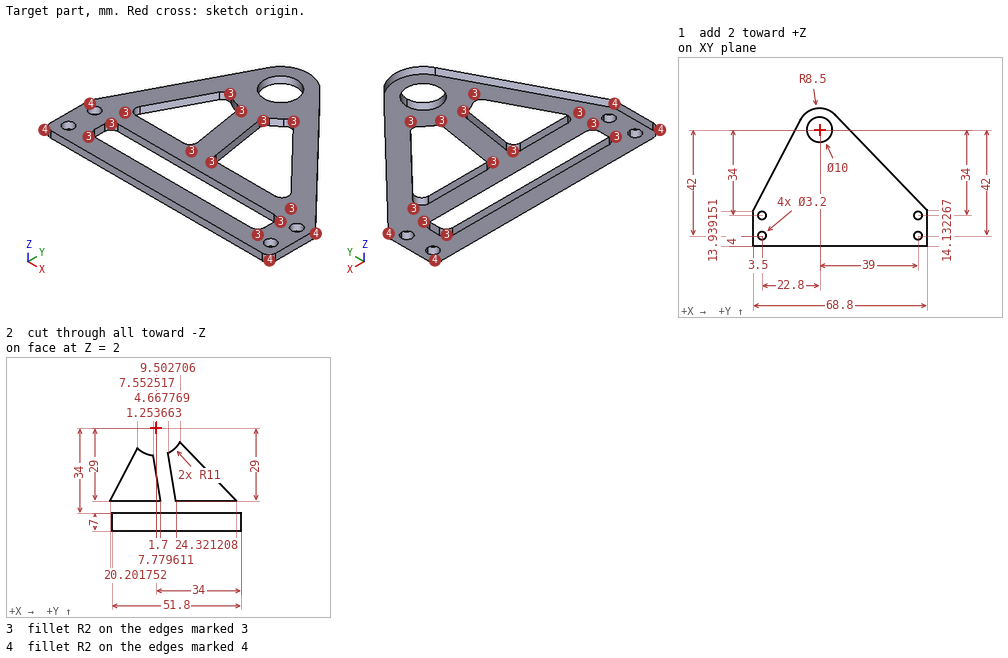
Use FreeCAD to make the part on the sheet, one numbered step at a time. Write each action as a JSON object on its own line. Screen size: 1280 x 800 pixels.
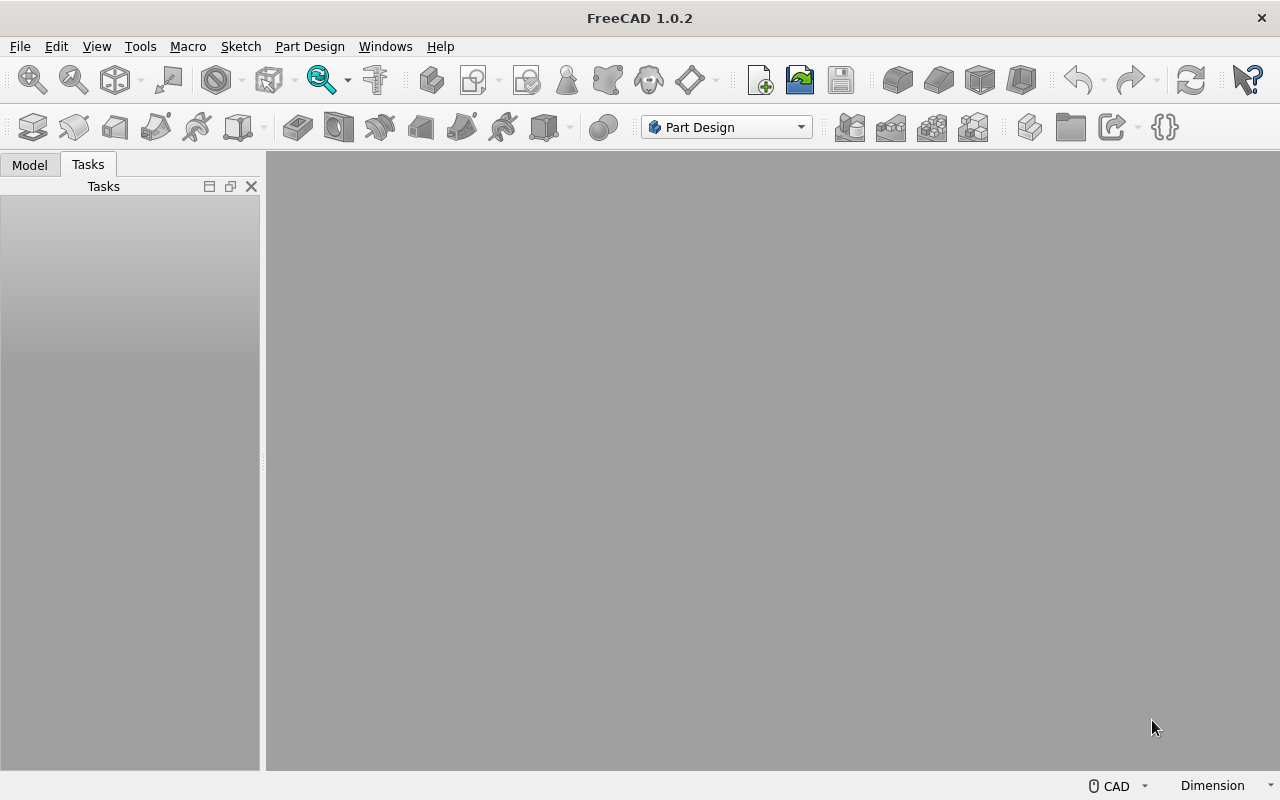
{"action": "left_click", "coordinate": [759, 80]}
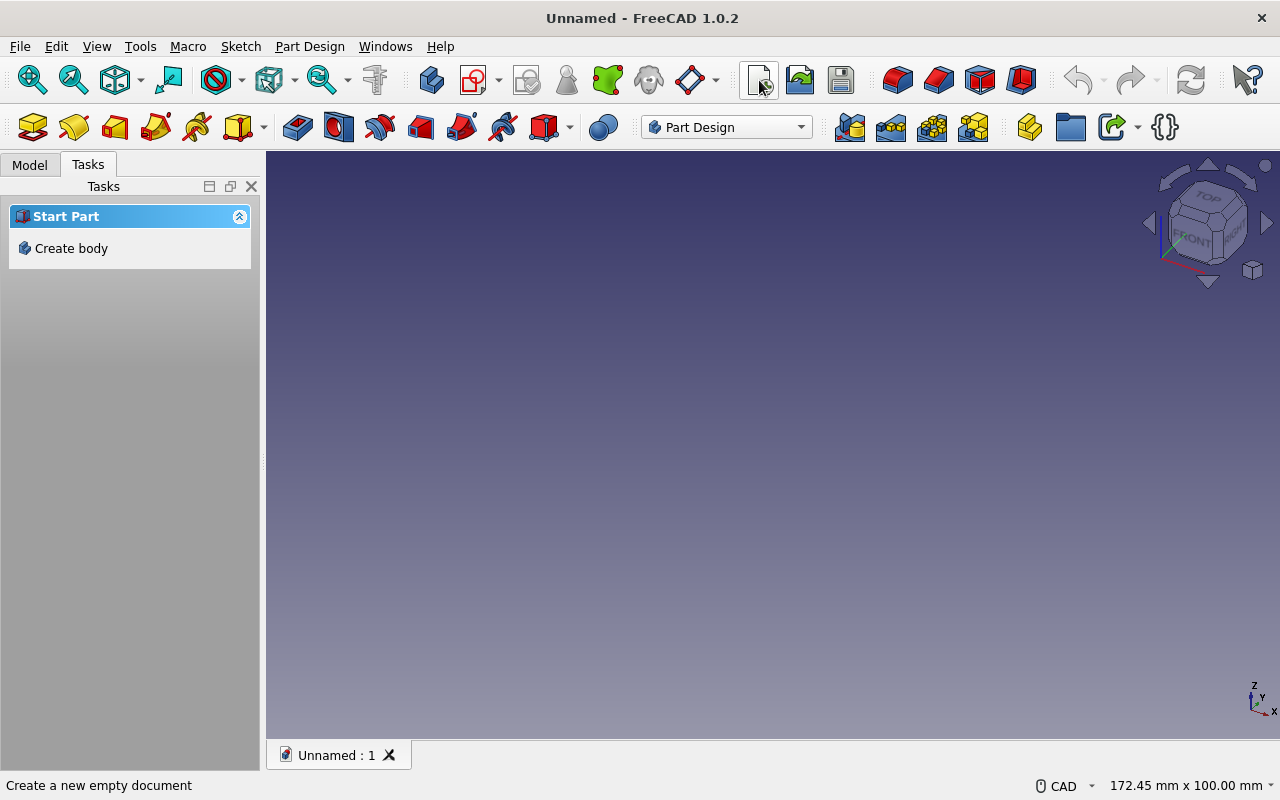
{"action": "left_click", "coordinate": [472, 80]}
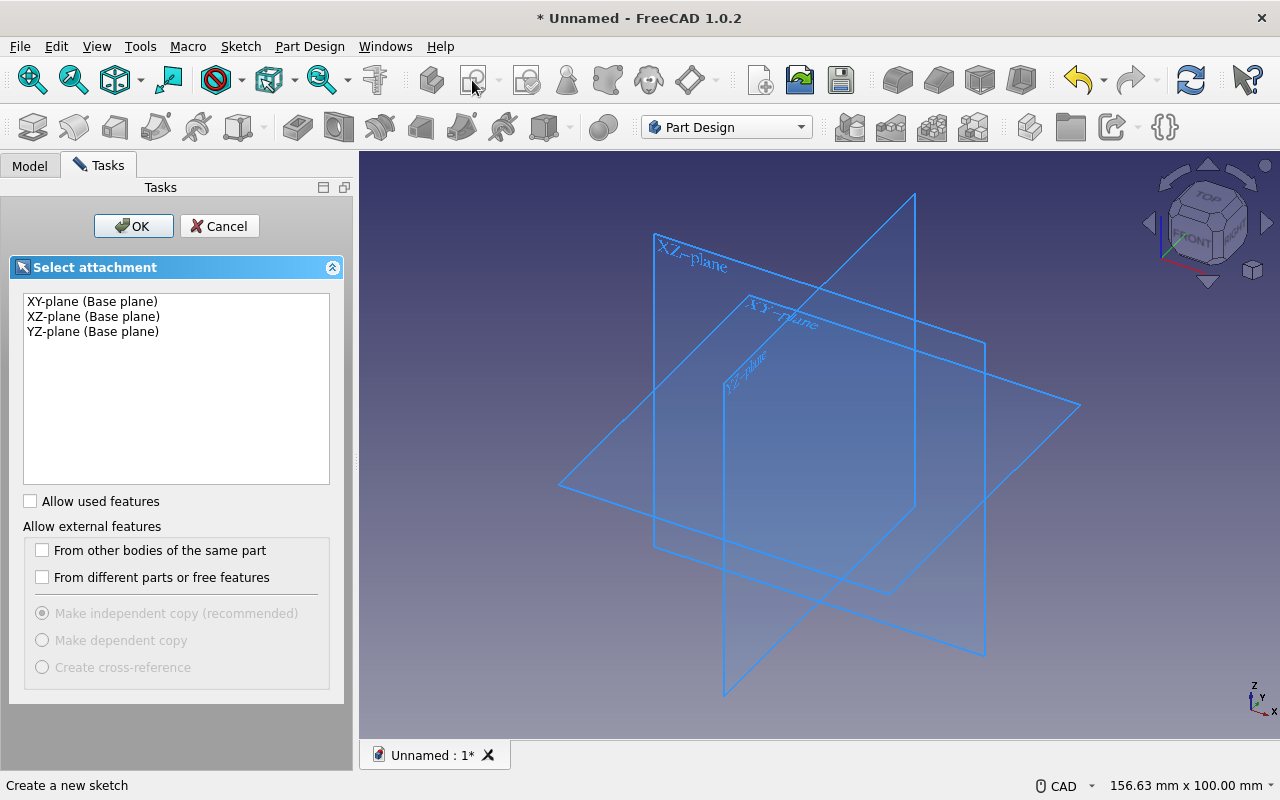
{"action": "left_click", "coordinate": [84, 302]}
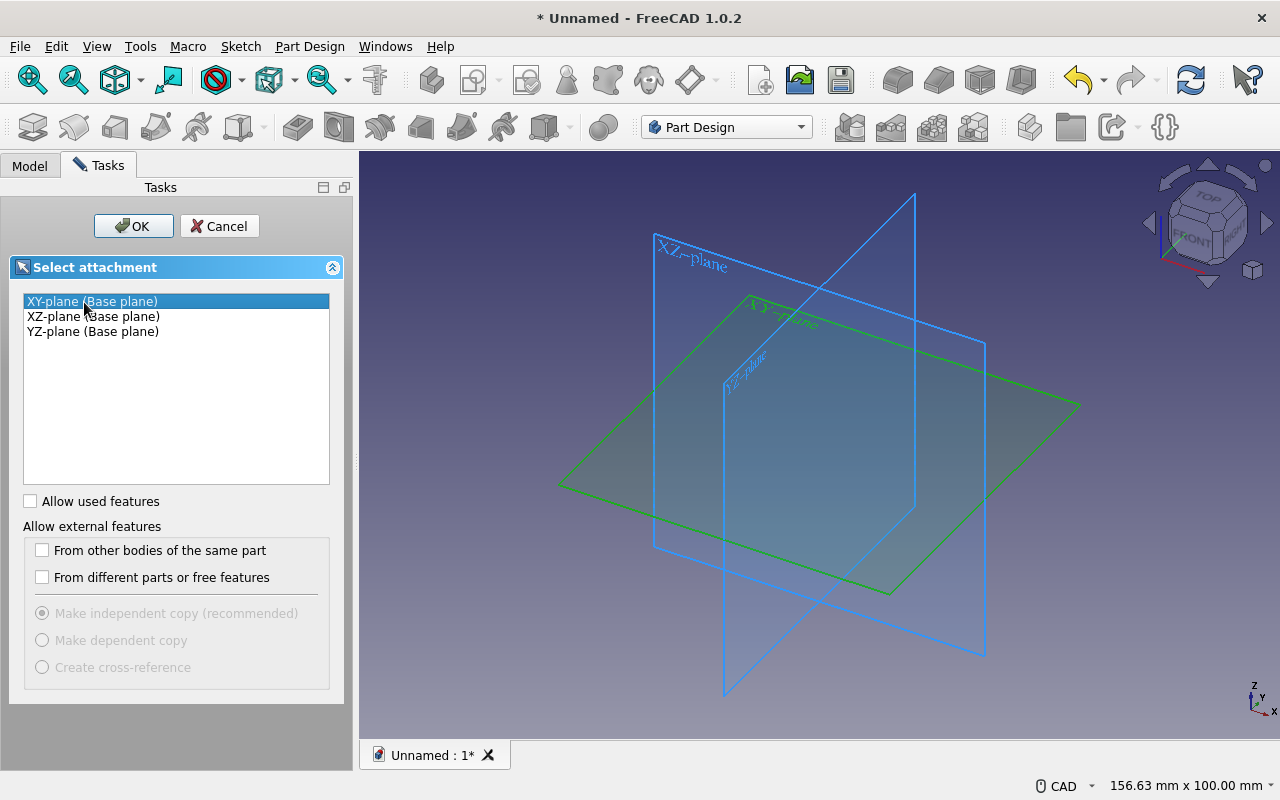
{"action": "left_click", "coordinate": [134, 226]}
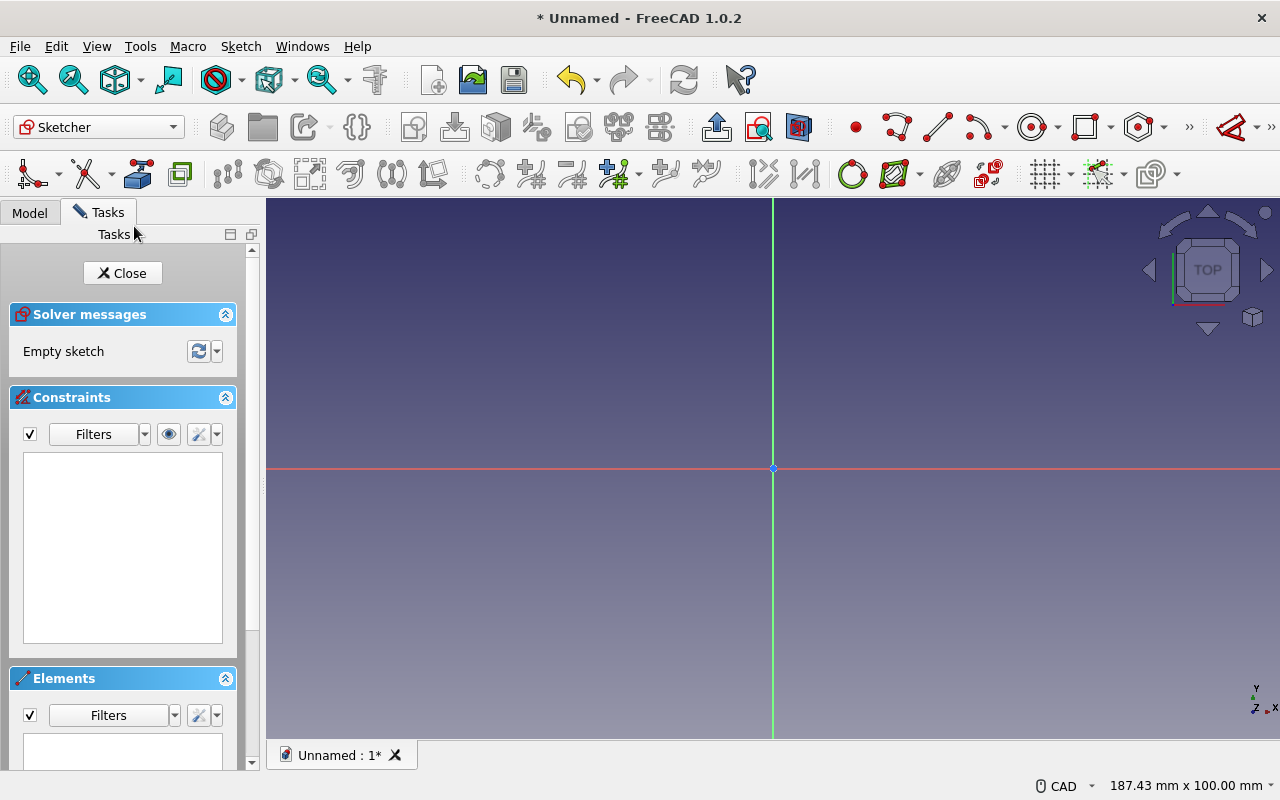
{"action": "scroll", "coordinate": [294, 226], "scroll_direction": "down", "scroll_amount": 1}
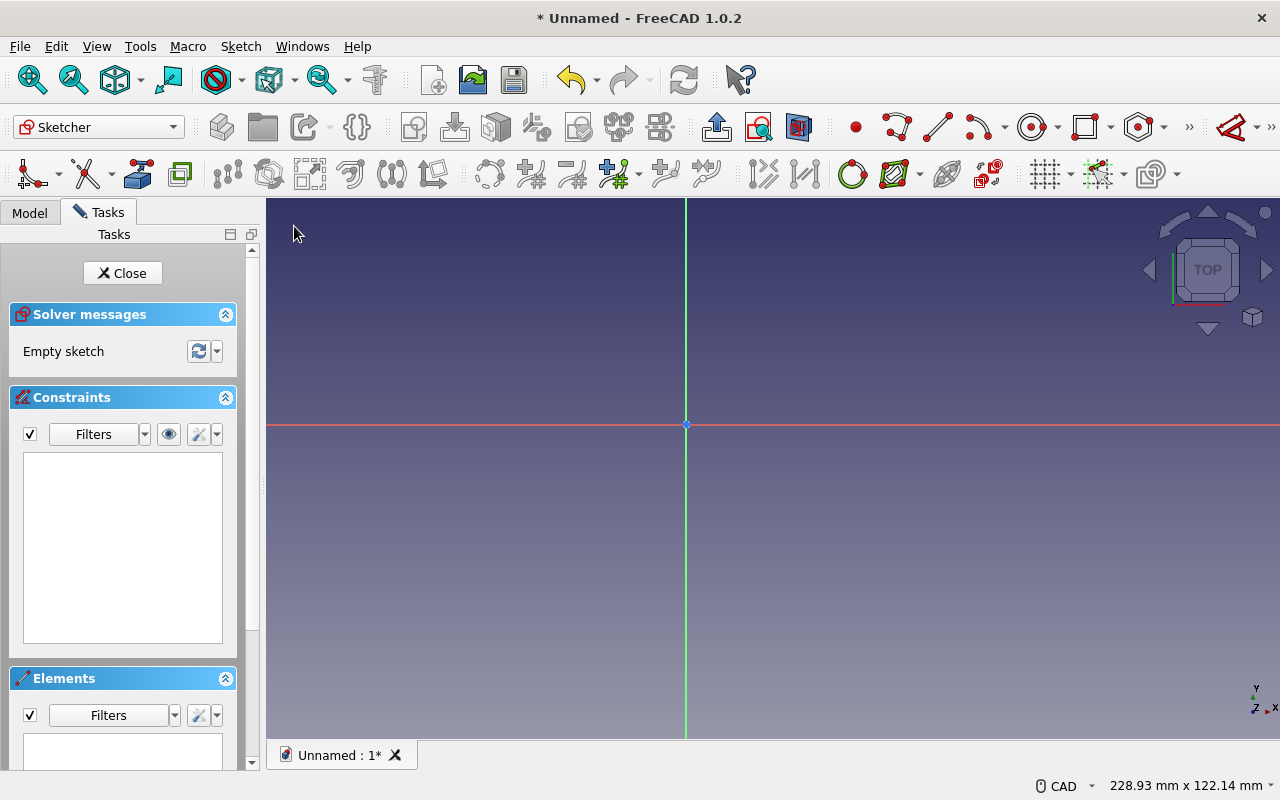
{"action": "scroll", "coordinate": [758, 588], "scroll_direction": "up", "scroll_amount": 2}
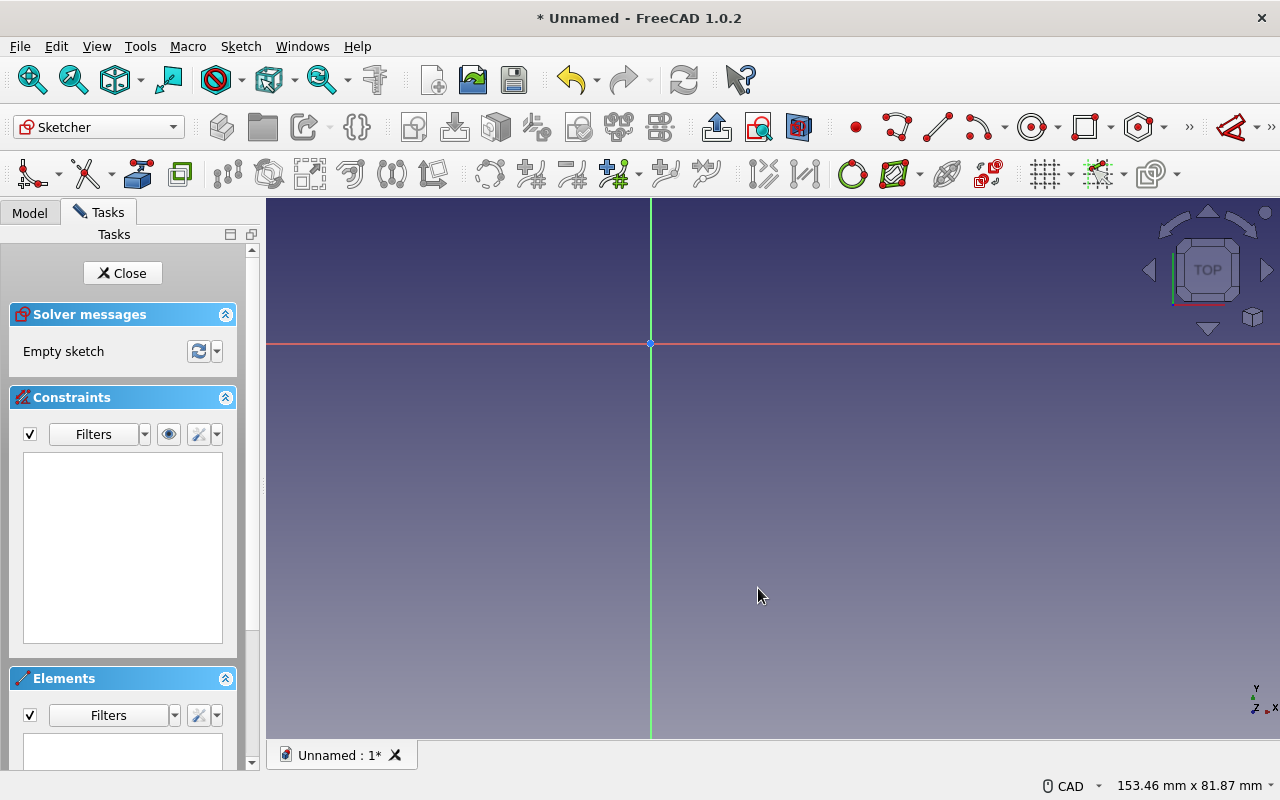
{"action": "key", "text": "g m"}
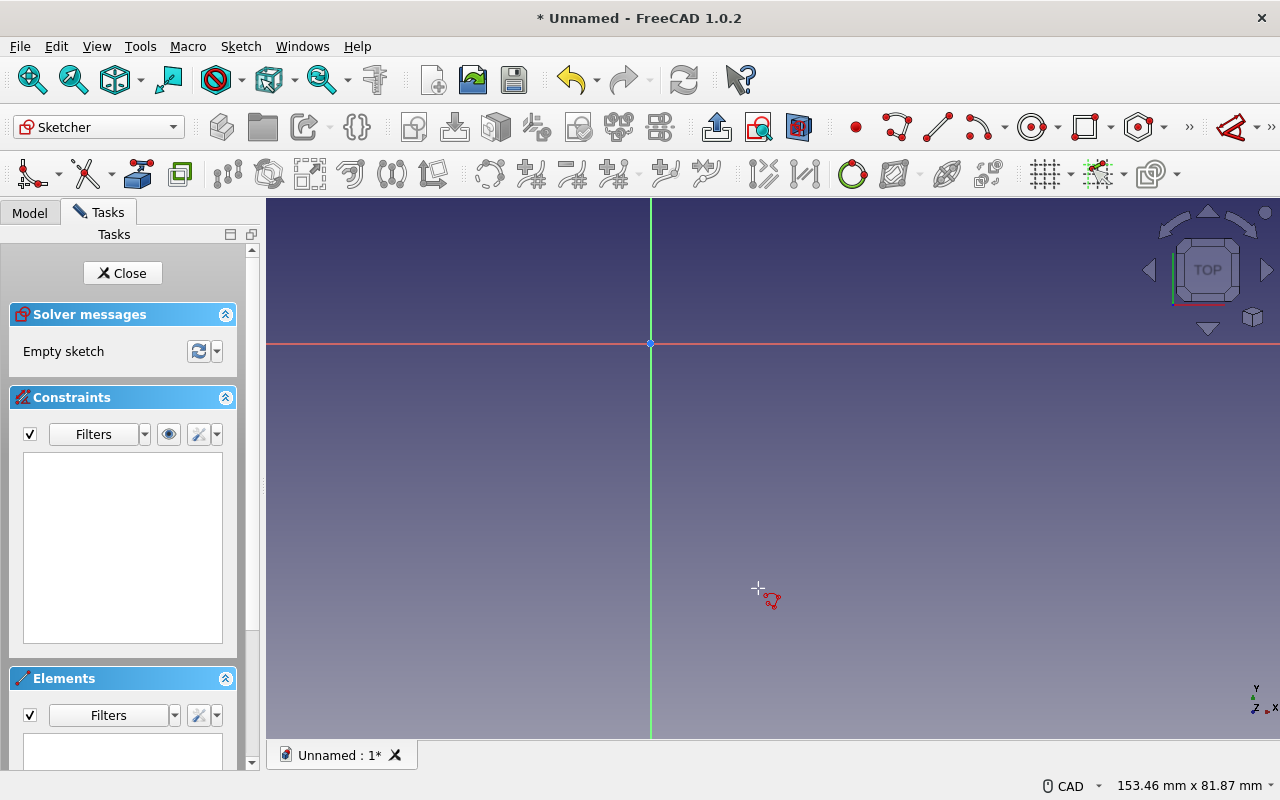
{"action": "left_click", "coordinate": [601, 318]}
{"action": "left_click", "coordinate": [477, 556]}
{"action": "left_click", "coordinate": [477, 648]}
{"action": "left_click", "coordinate": [931, 648]}
{"action": "left_click", "coordinate": [931, 554]}
{"action": "left_click", "coordinate": [691, 305]}
{"action": "right_click", "coordinate": [691, 305]}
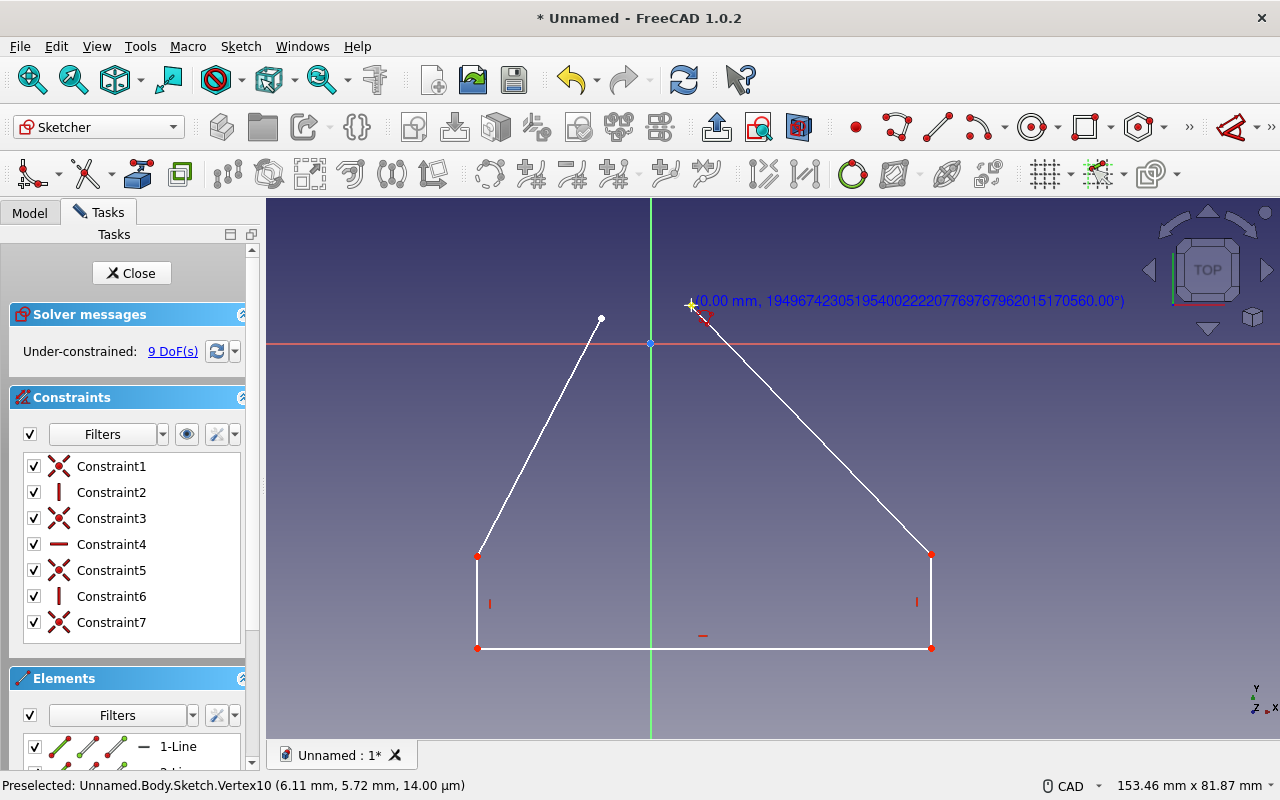
{"action": "key", "text": "g 3 a"}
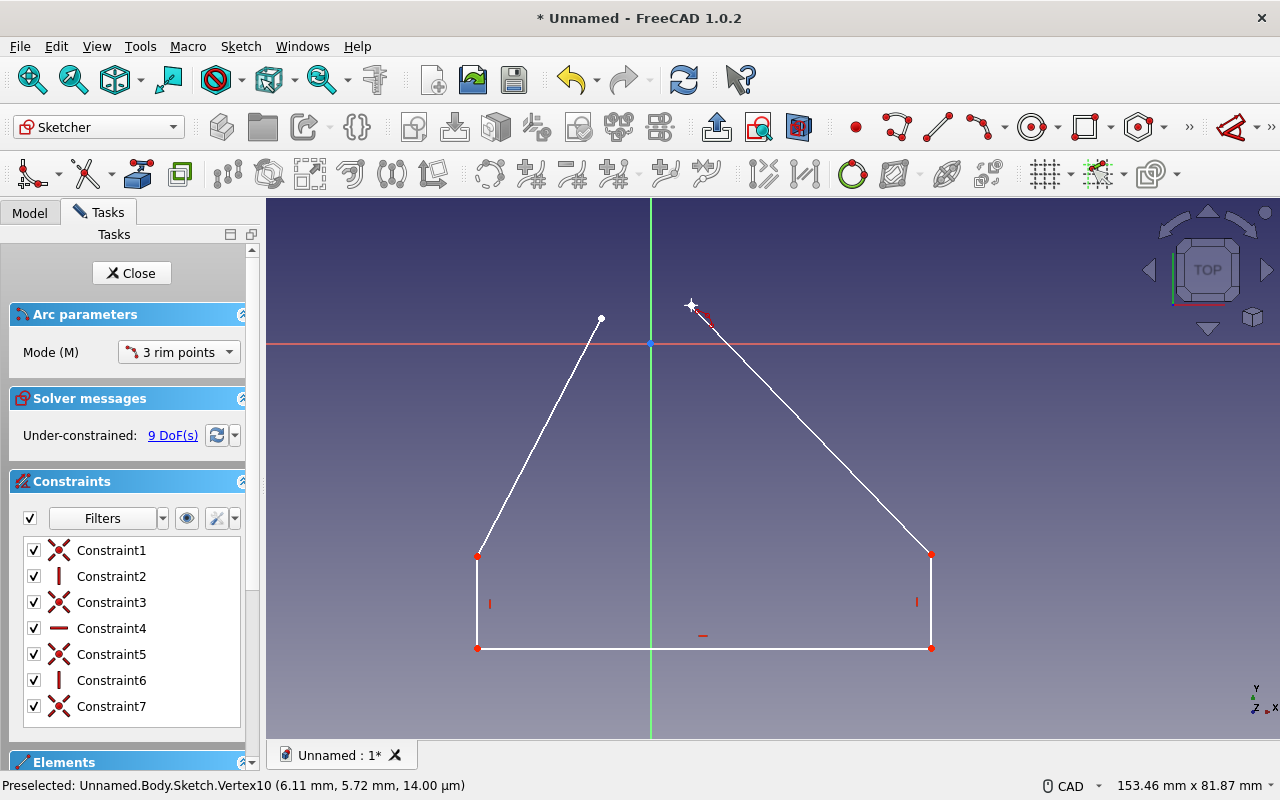
{"action": "left_click", "coordinate": [691, 306]}
{"action": "left_click", "coordinate": [601, 319]}
{"action": "left_click", "coordinate": [632, 291]}